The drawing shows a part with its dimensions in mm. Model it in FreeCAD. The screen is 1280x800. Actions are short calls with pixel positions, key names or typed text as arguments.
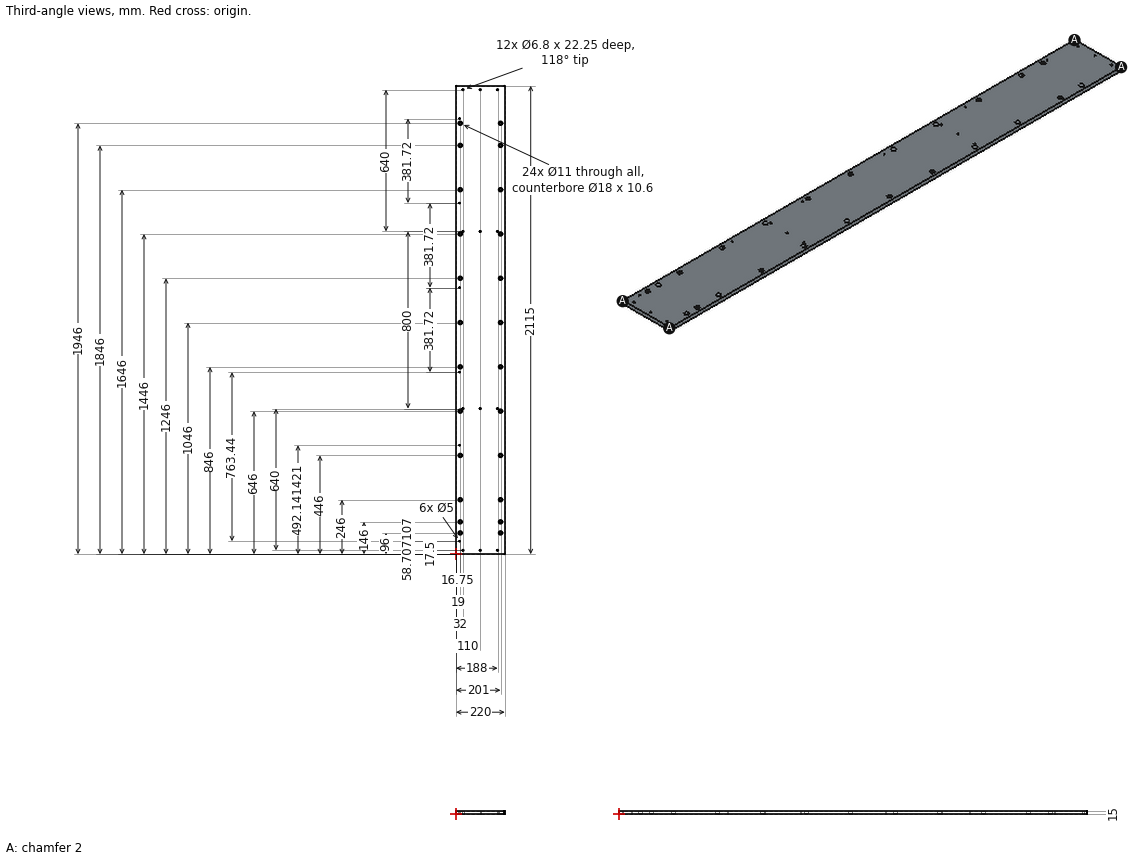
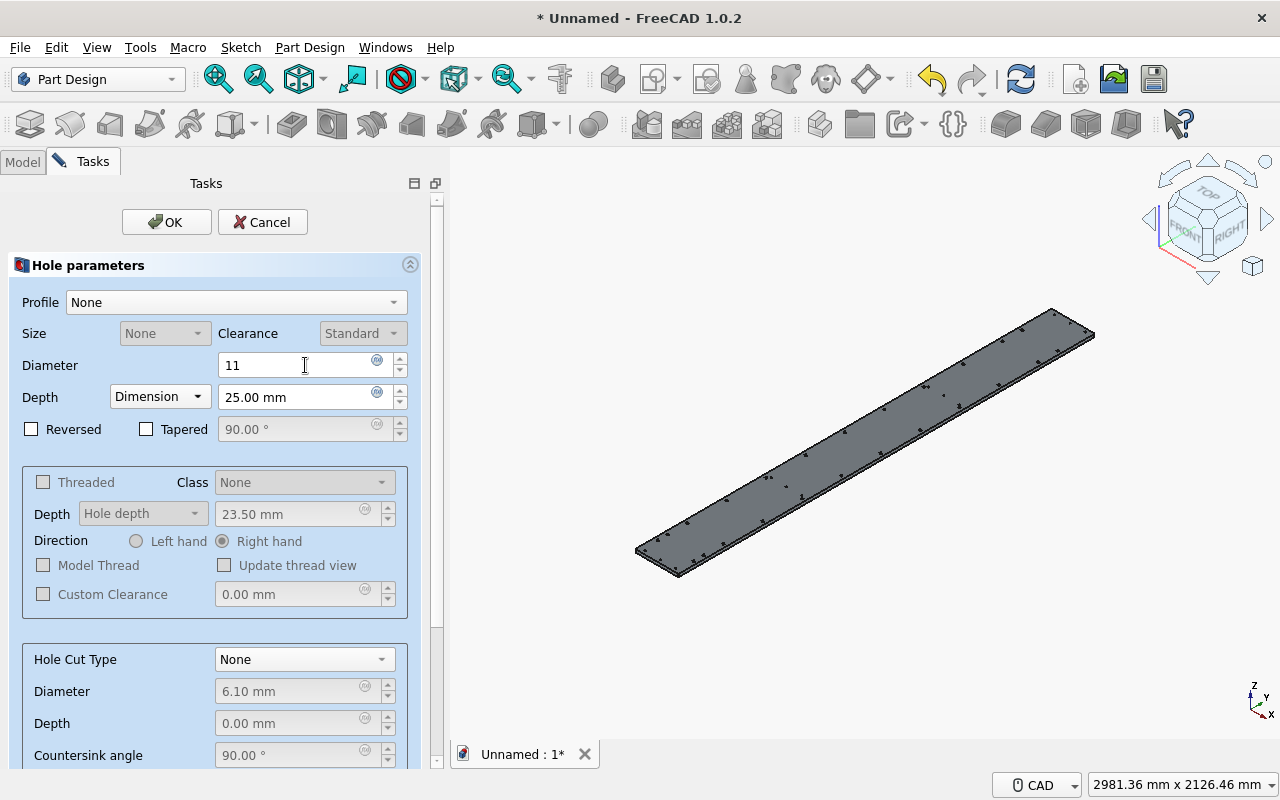
click(161, 396)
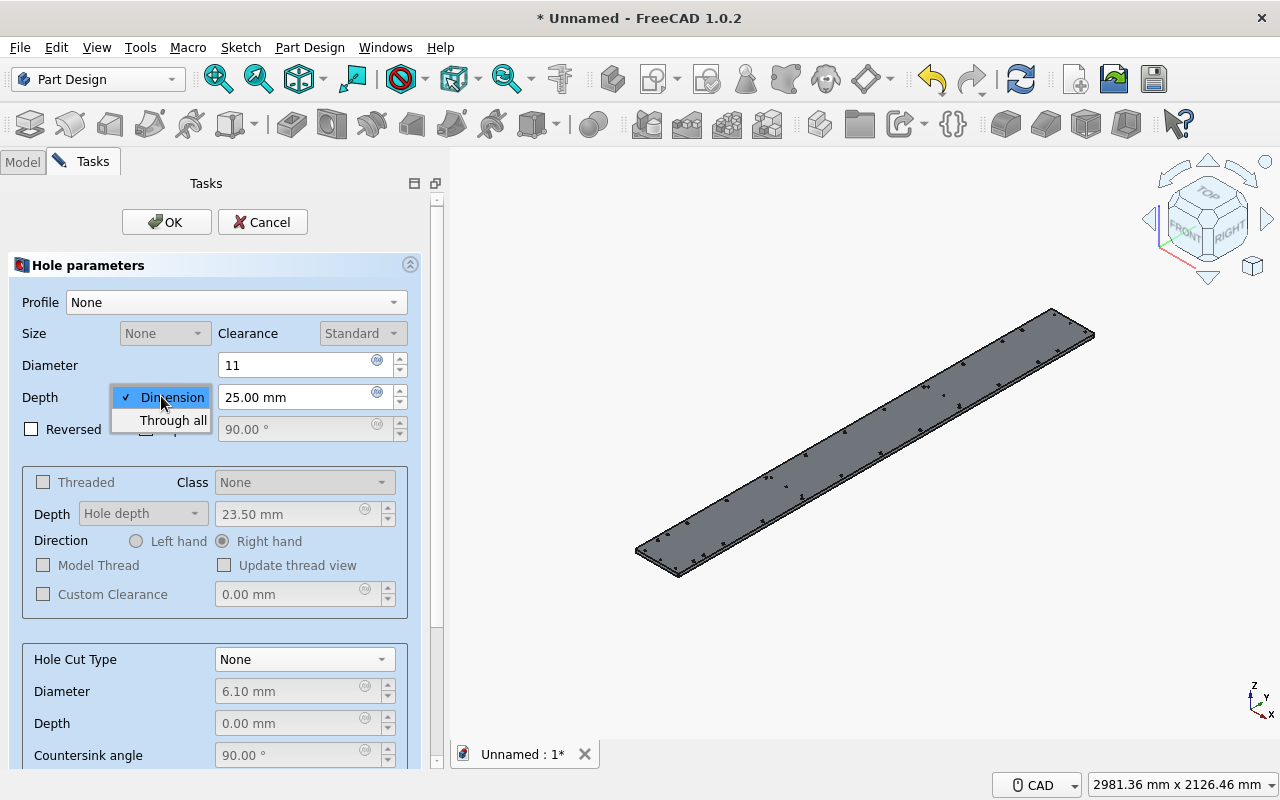
click(160, 420)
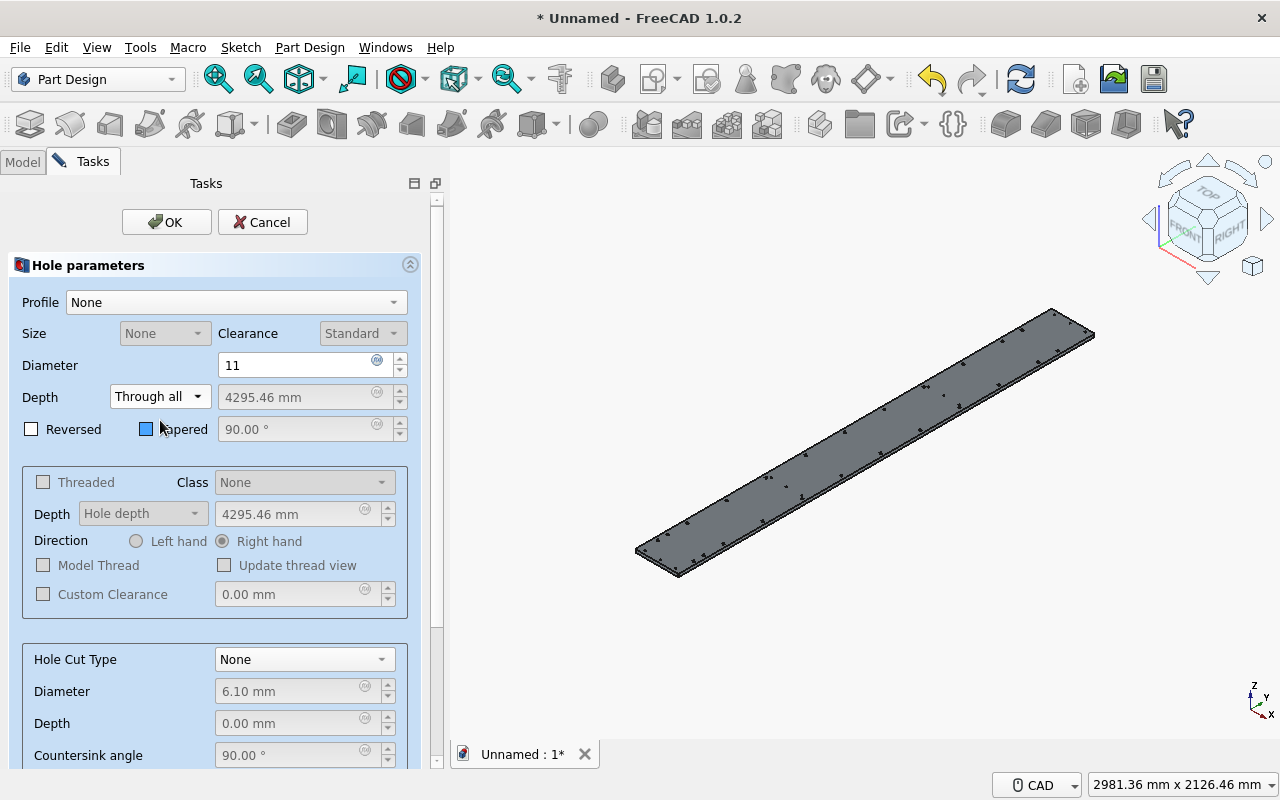
click(306, 660)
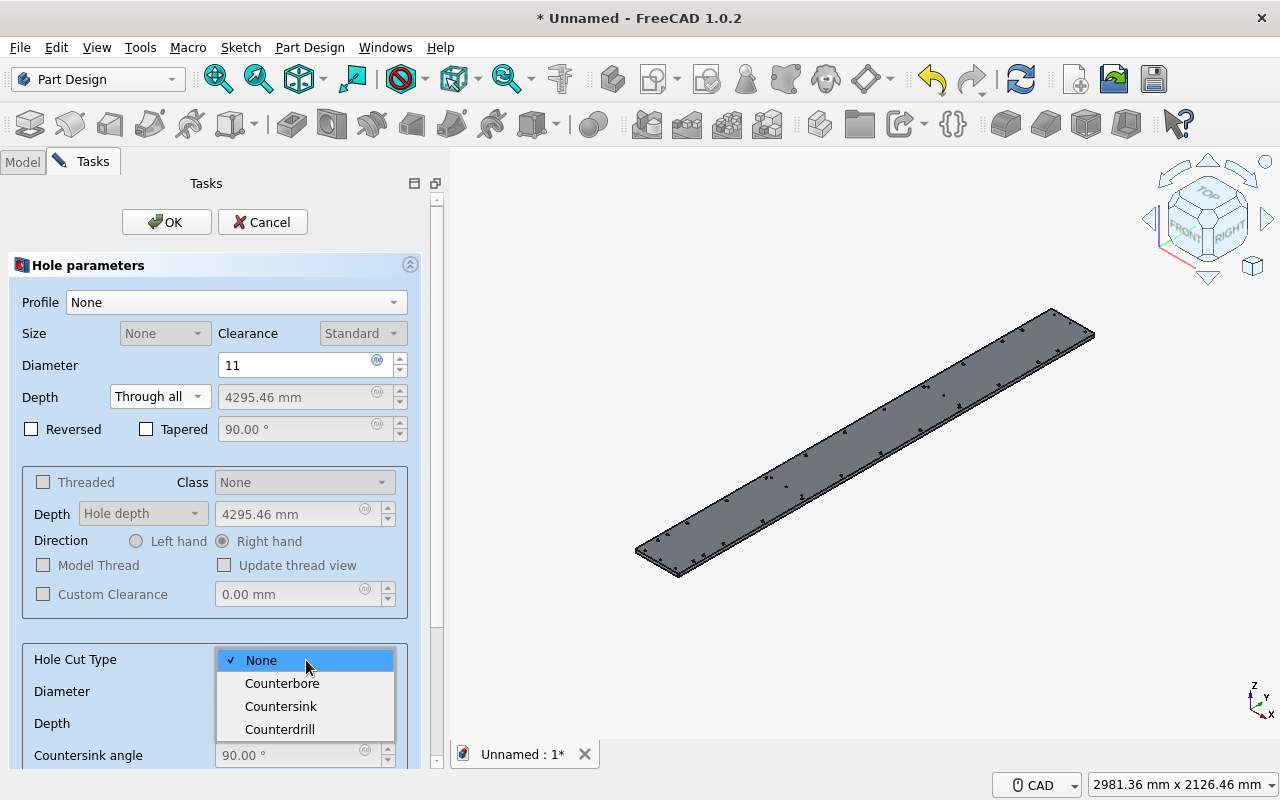
click(304, 684)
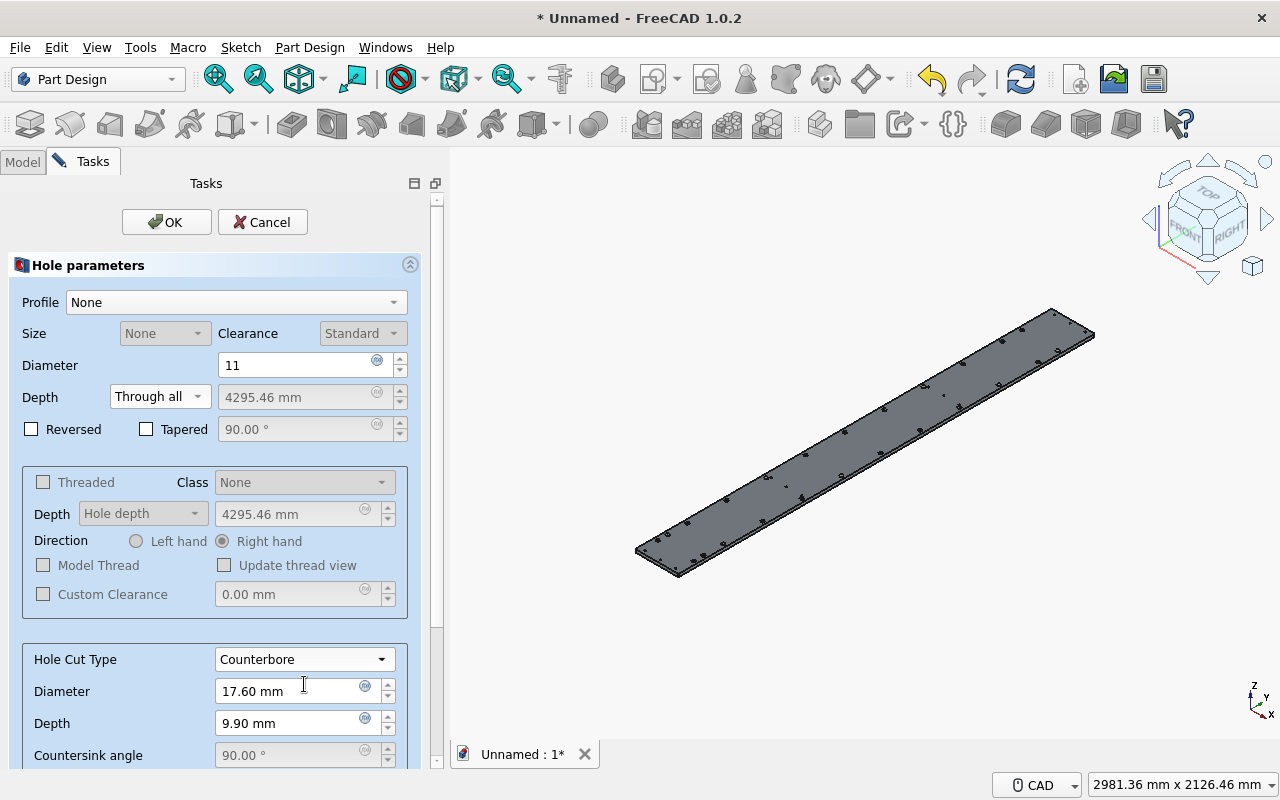
triple_click(298, 691)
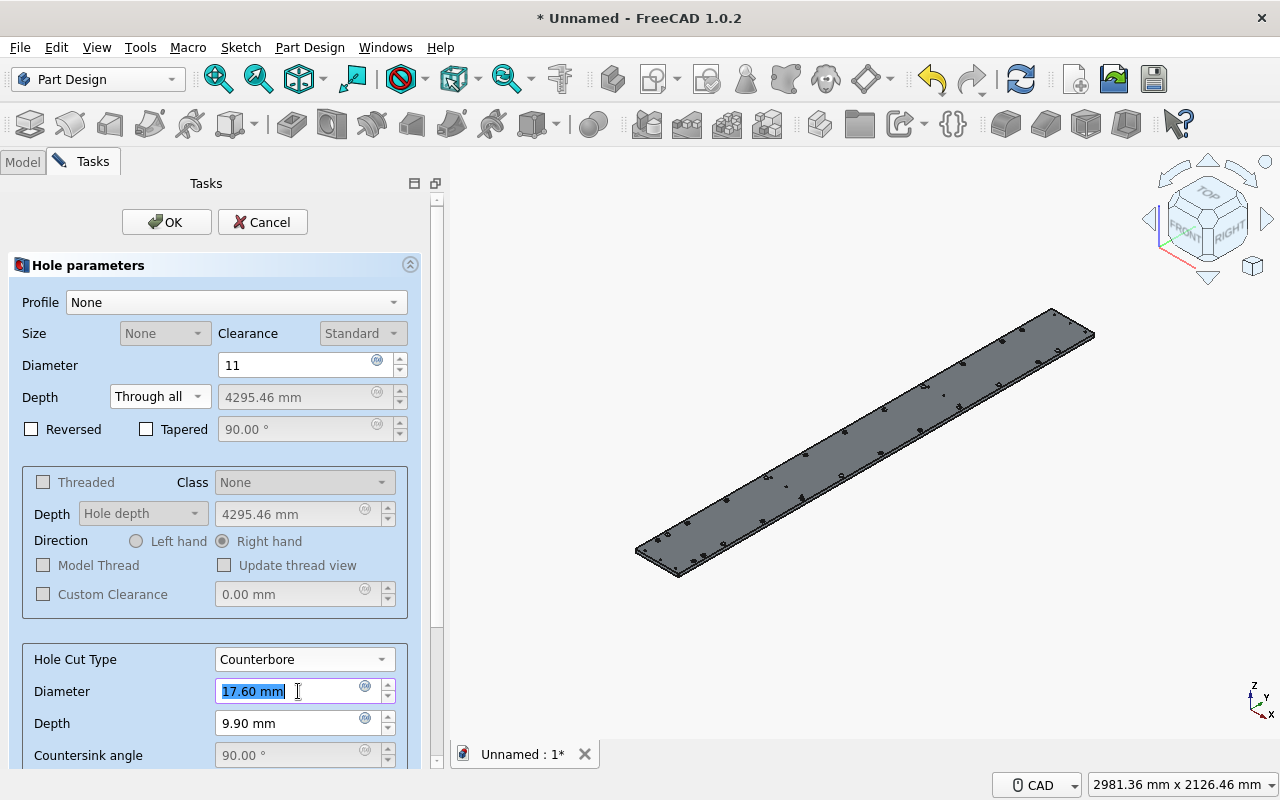
text(18)
key(Tab)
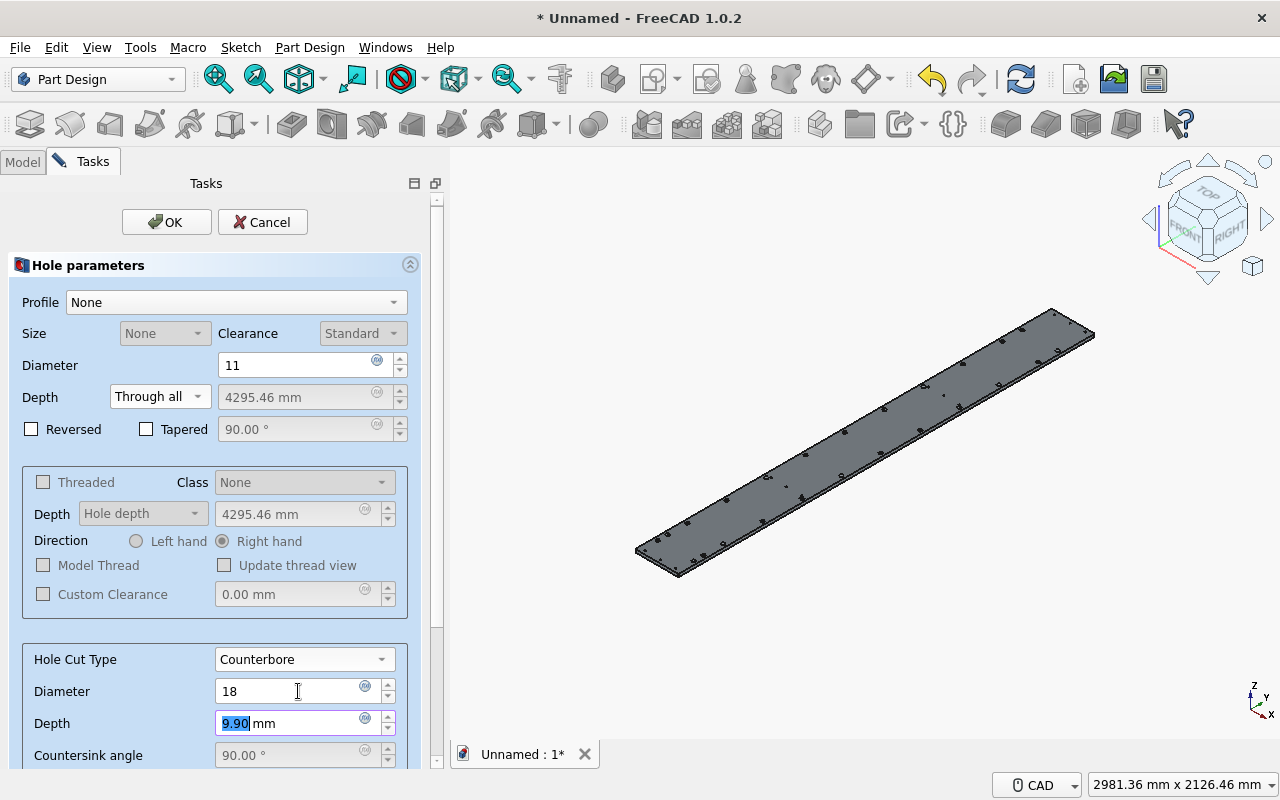
text(10.6)
key(Tab)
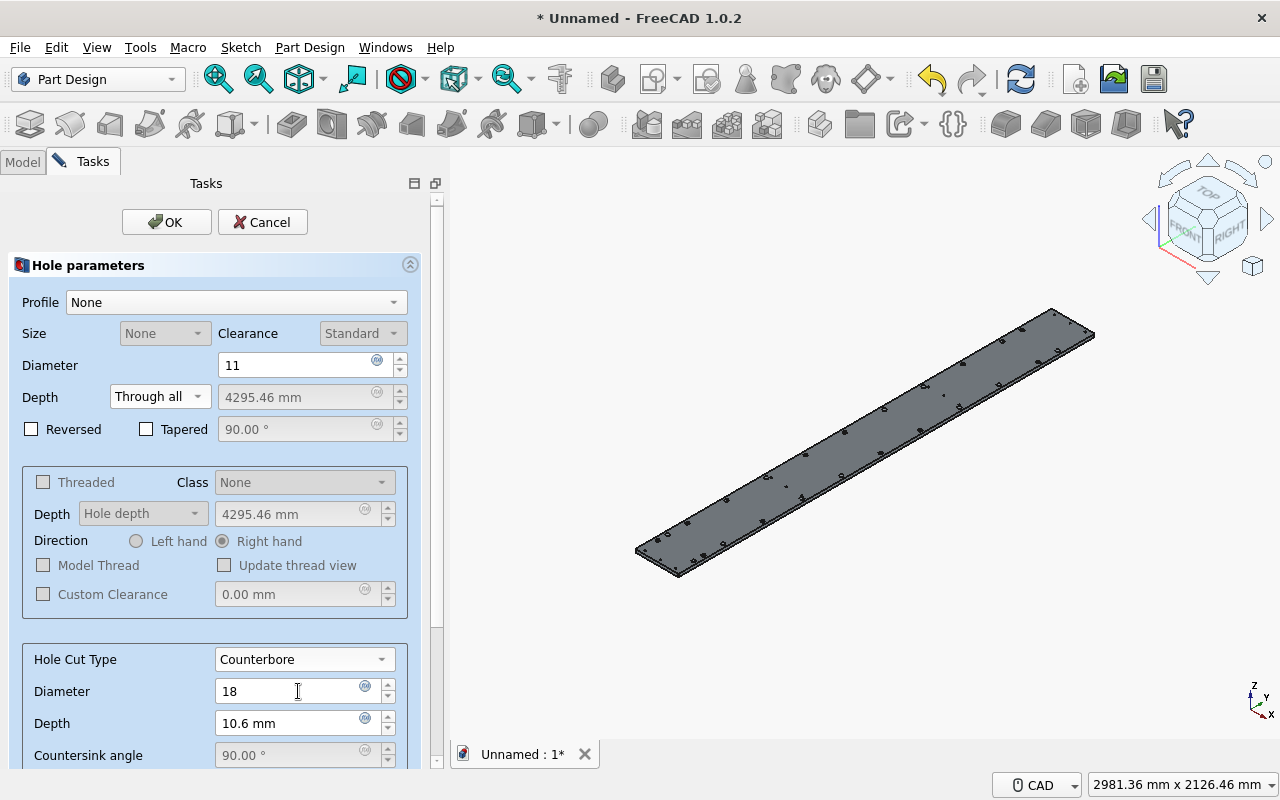
click(167, 222)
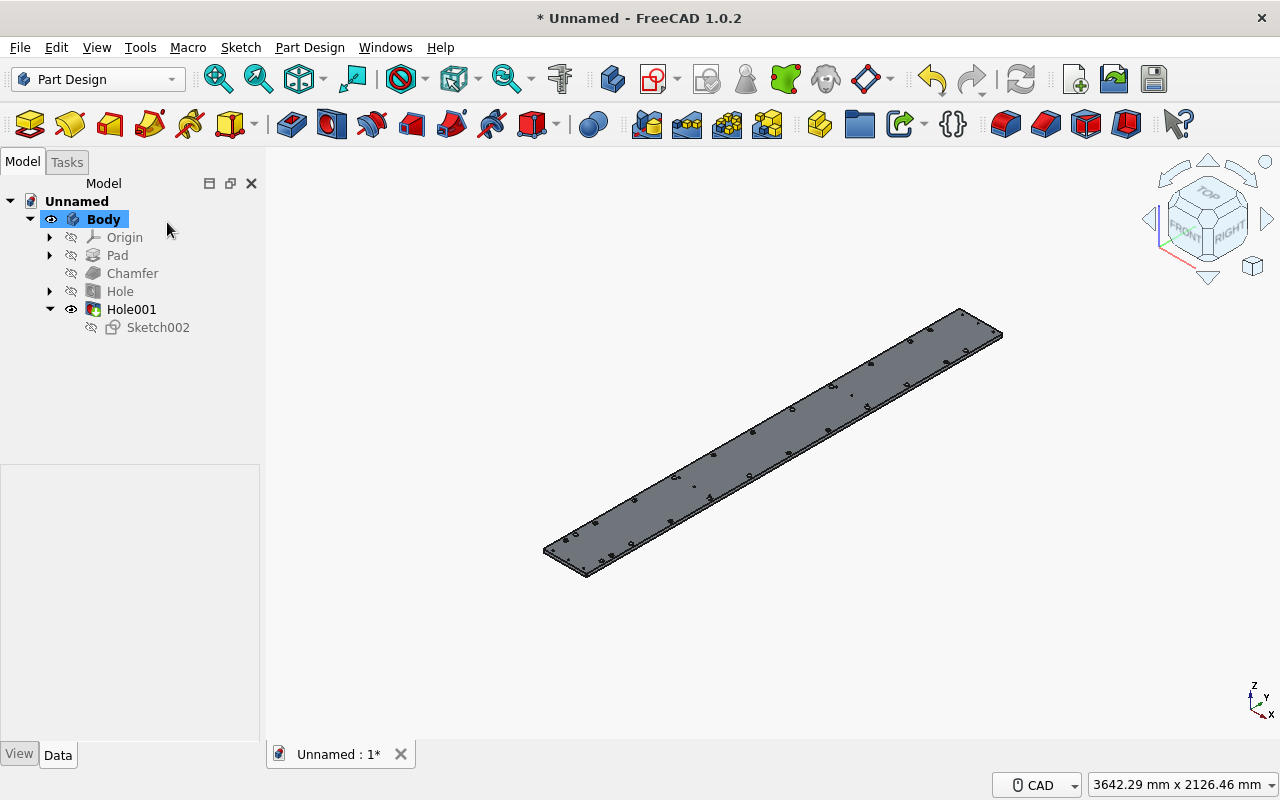
click(714, 475)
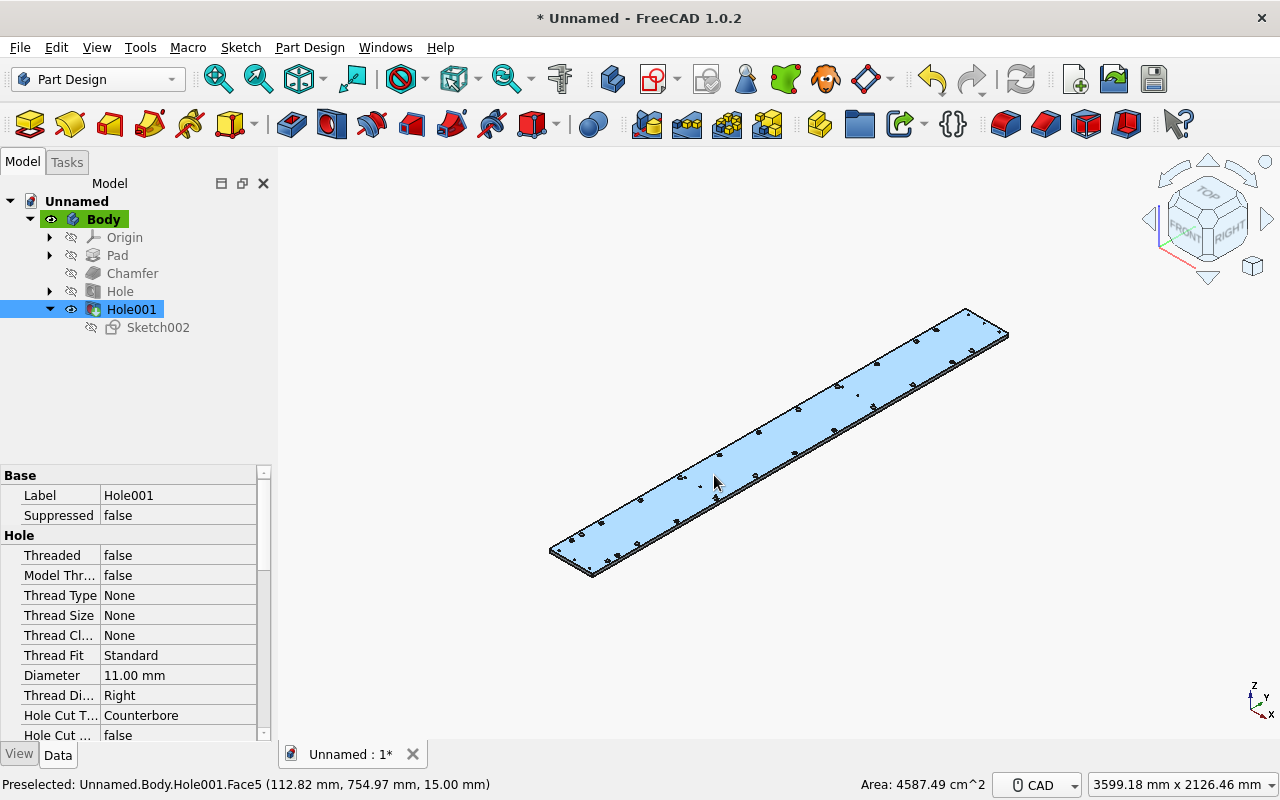
click(654, 80)